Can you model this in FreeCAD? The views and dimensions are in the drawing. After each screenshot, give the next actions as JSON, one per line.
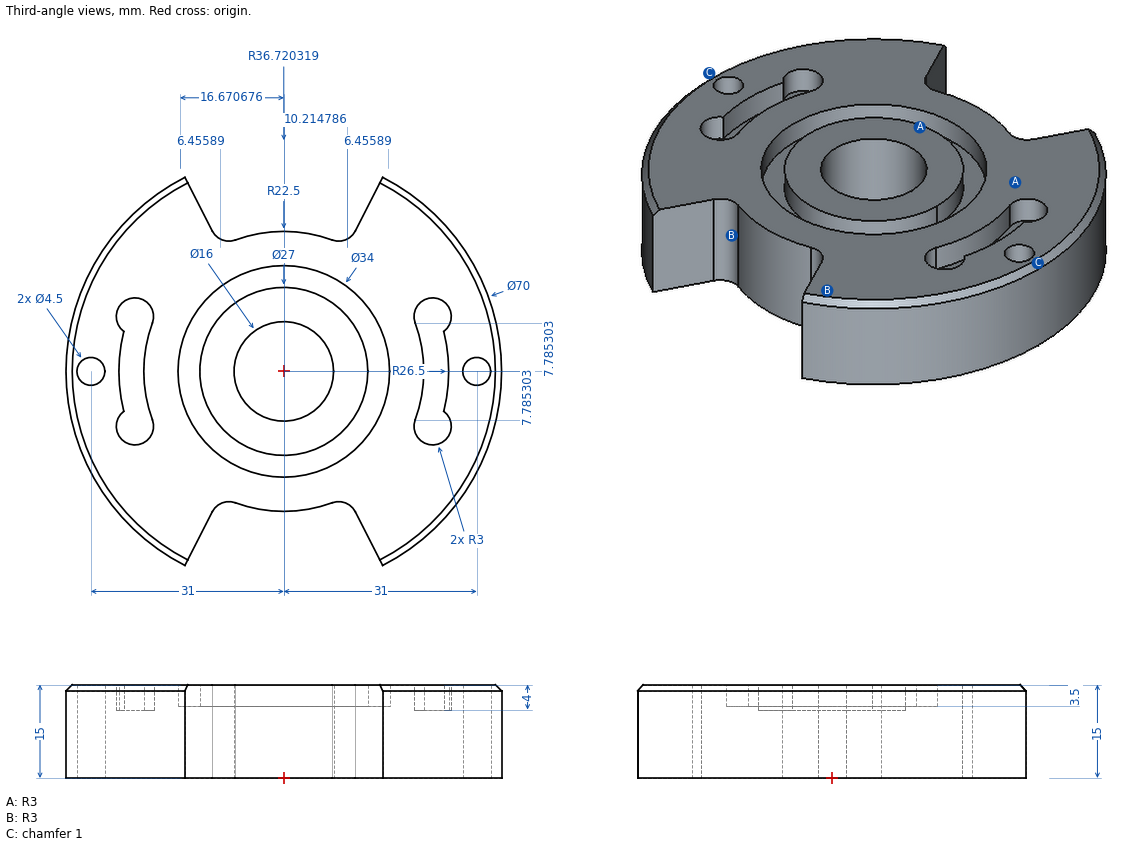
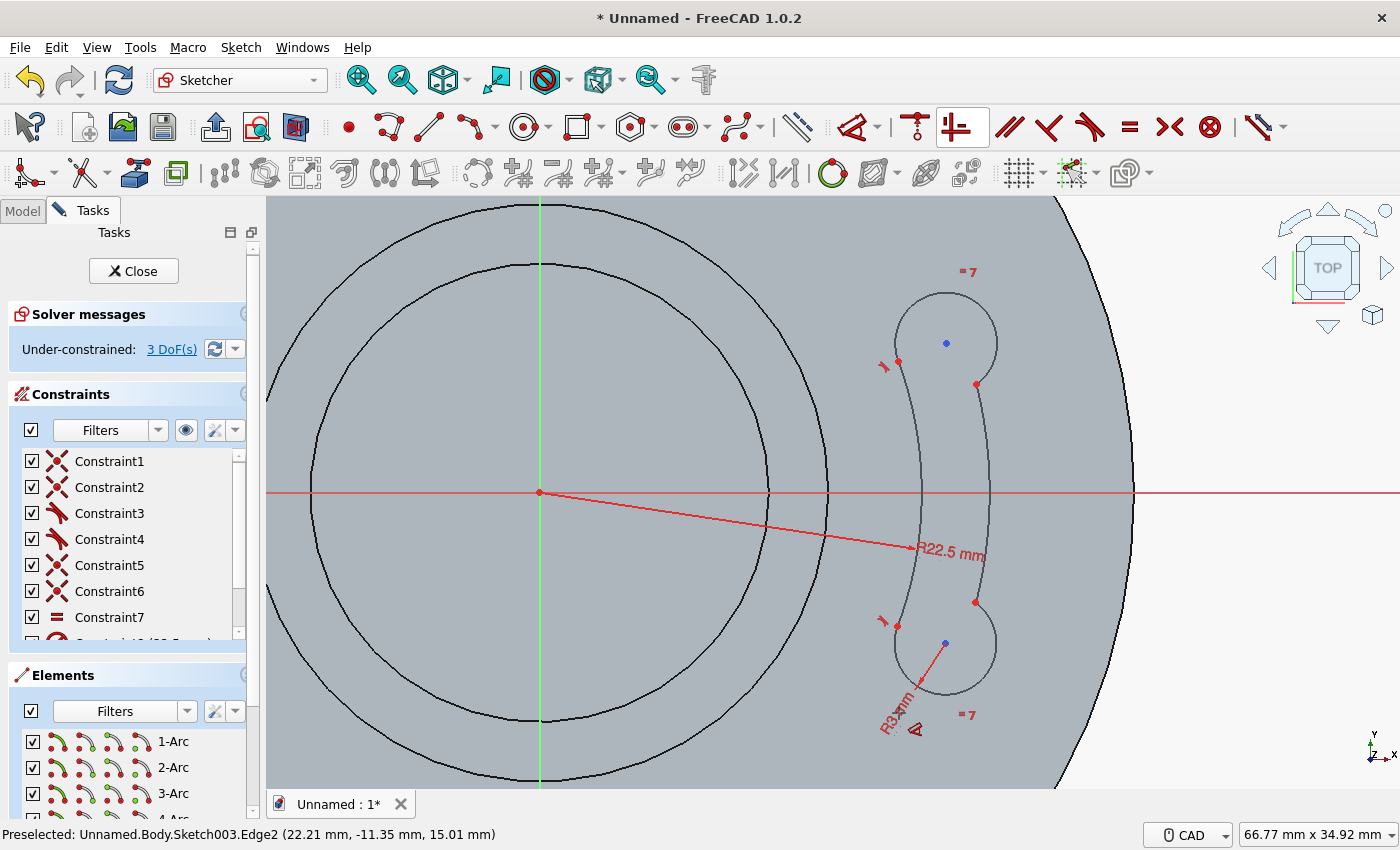
{"action": "left_click", "coordinate": [987, 538]}
{"action": "left_click", "coordinate": [1042, 544]}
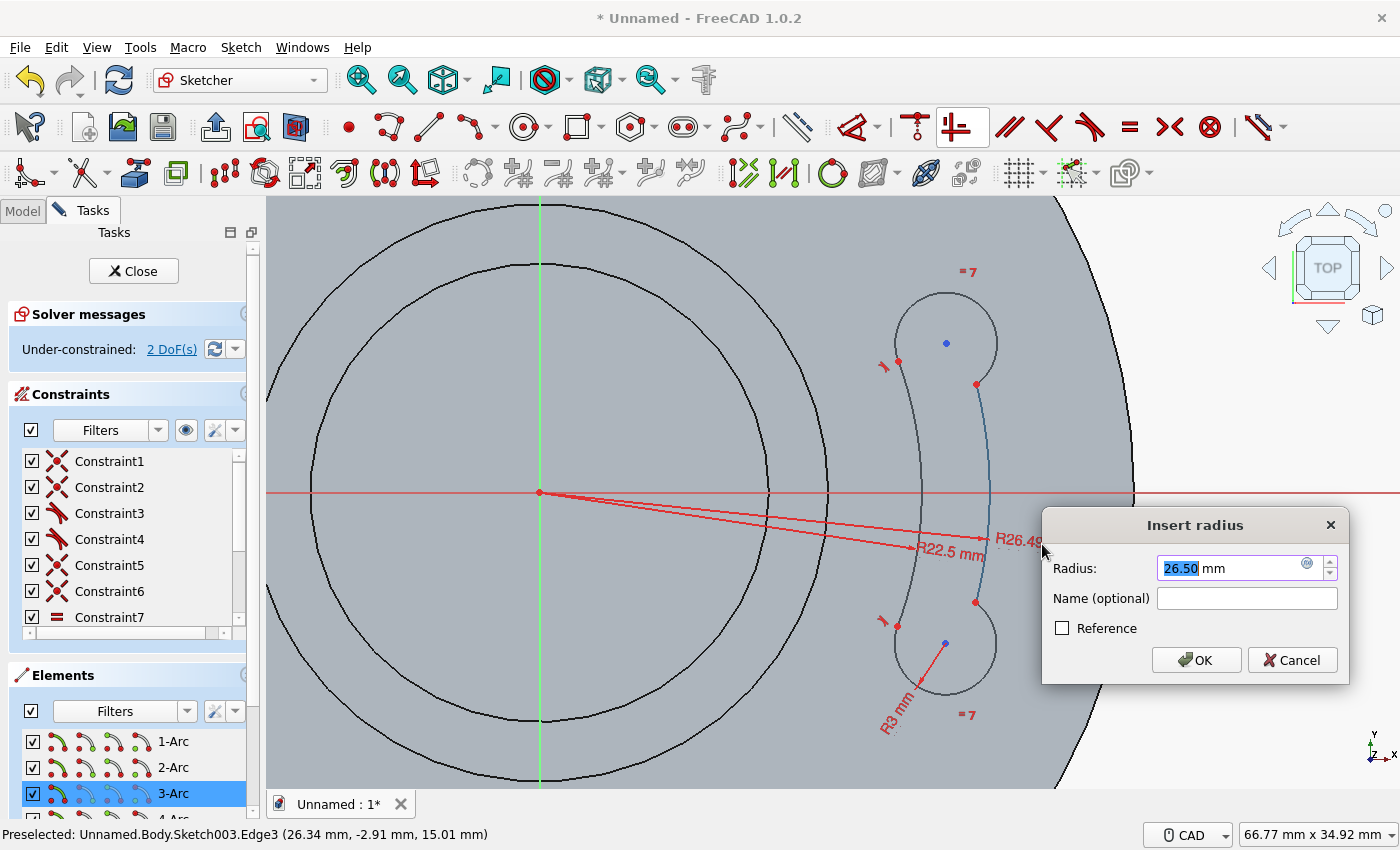
{"action": "type", "text": "26.5"}
{"action": "key", "text": "Return"}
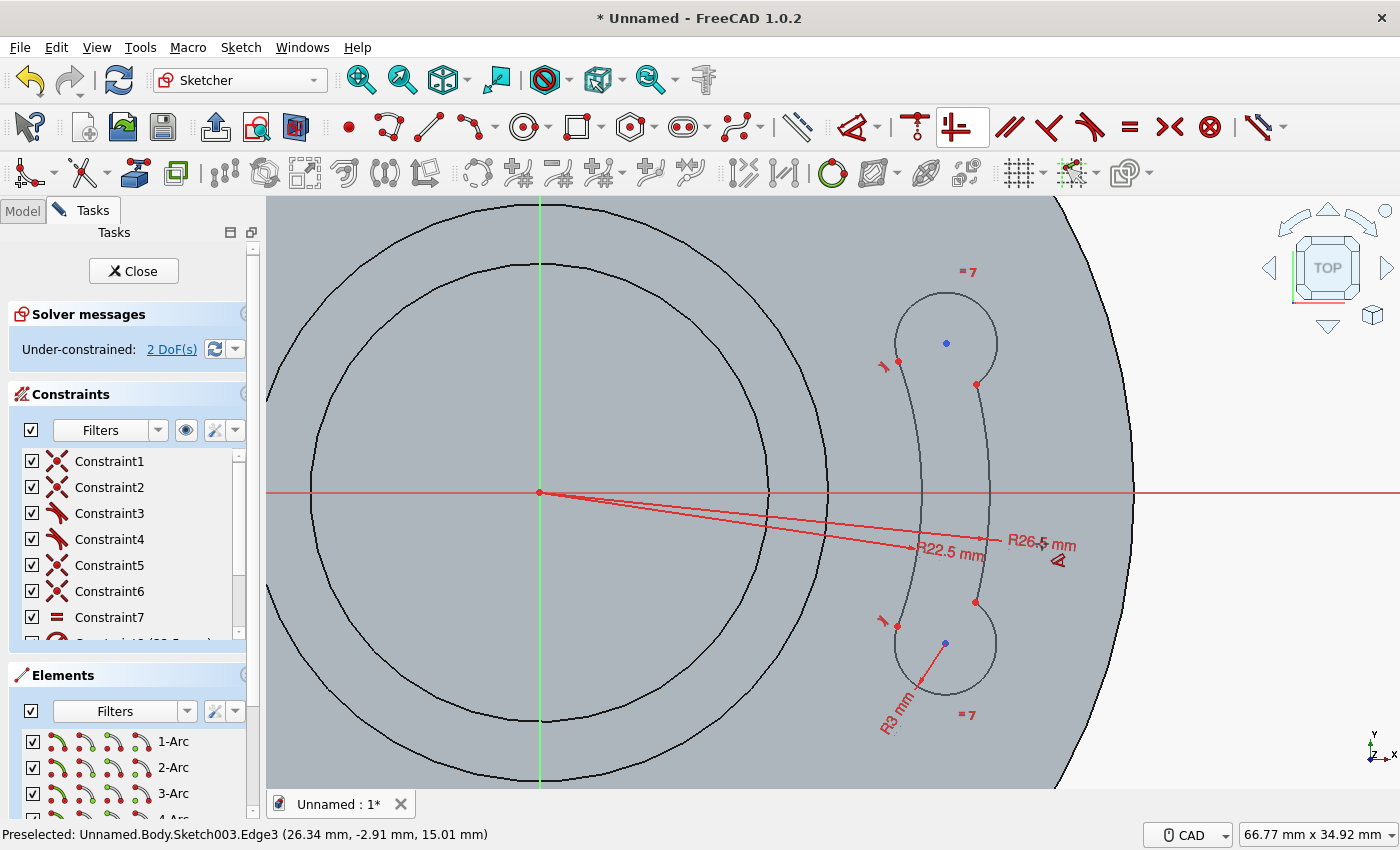
{"action": "left_click", "coordinate": [898, 626]}
{"action": "left_click", "coordinate": [506, 559]}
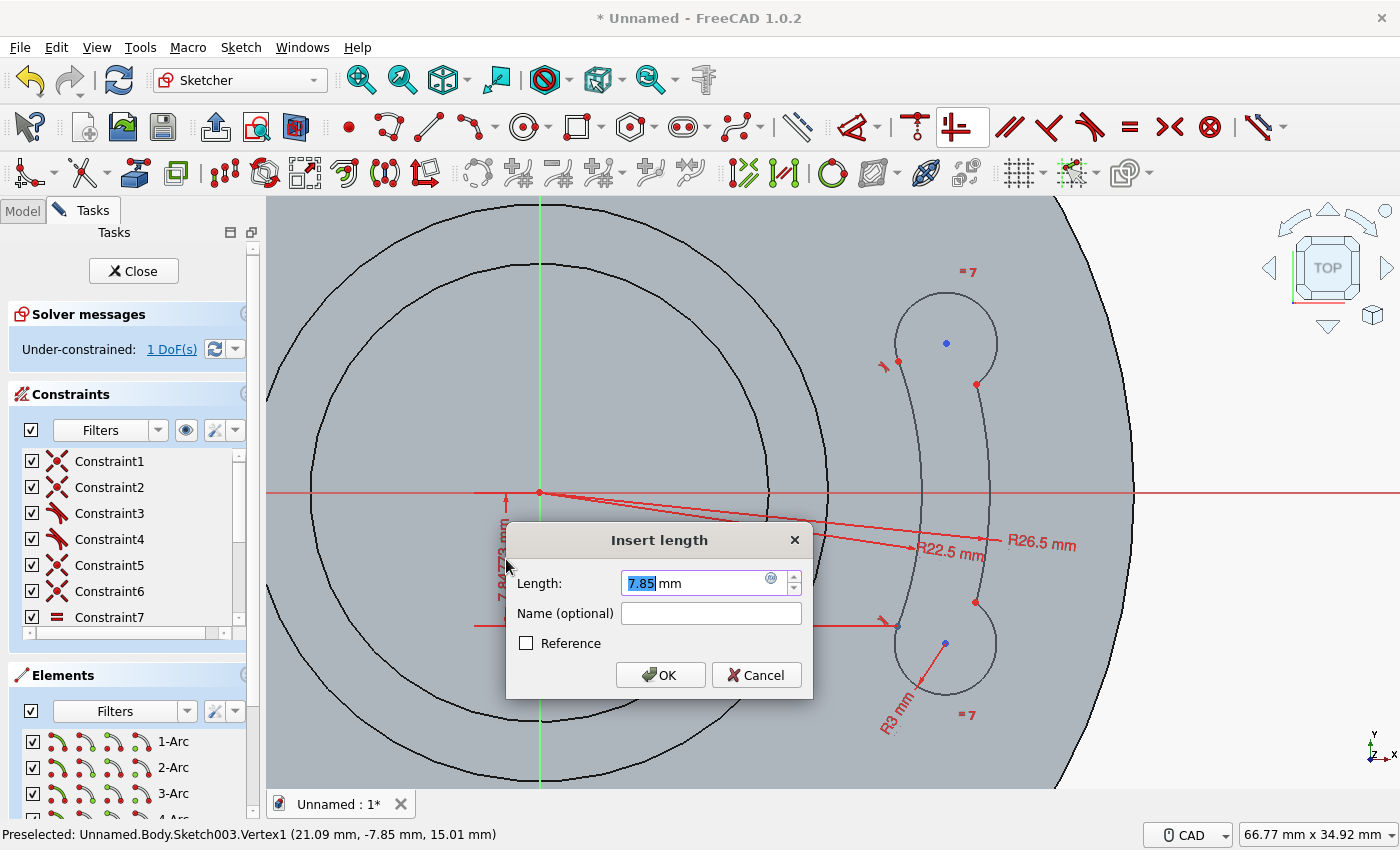
{"action": "type", "text": "7.785303"}
{"action": "key", "text": "Return"}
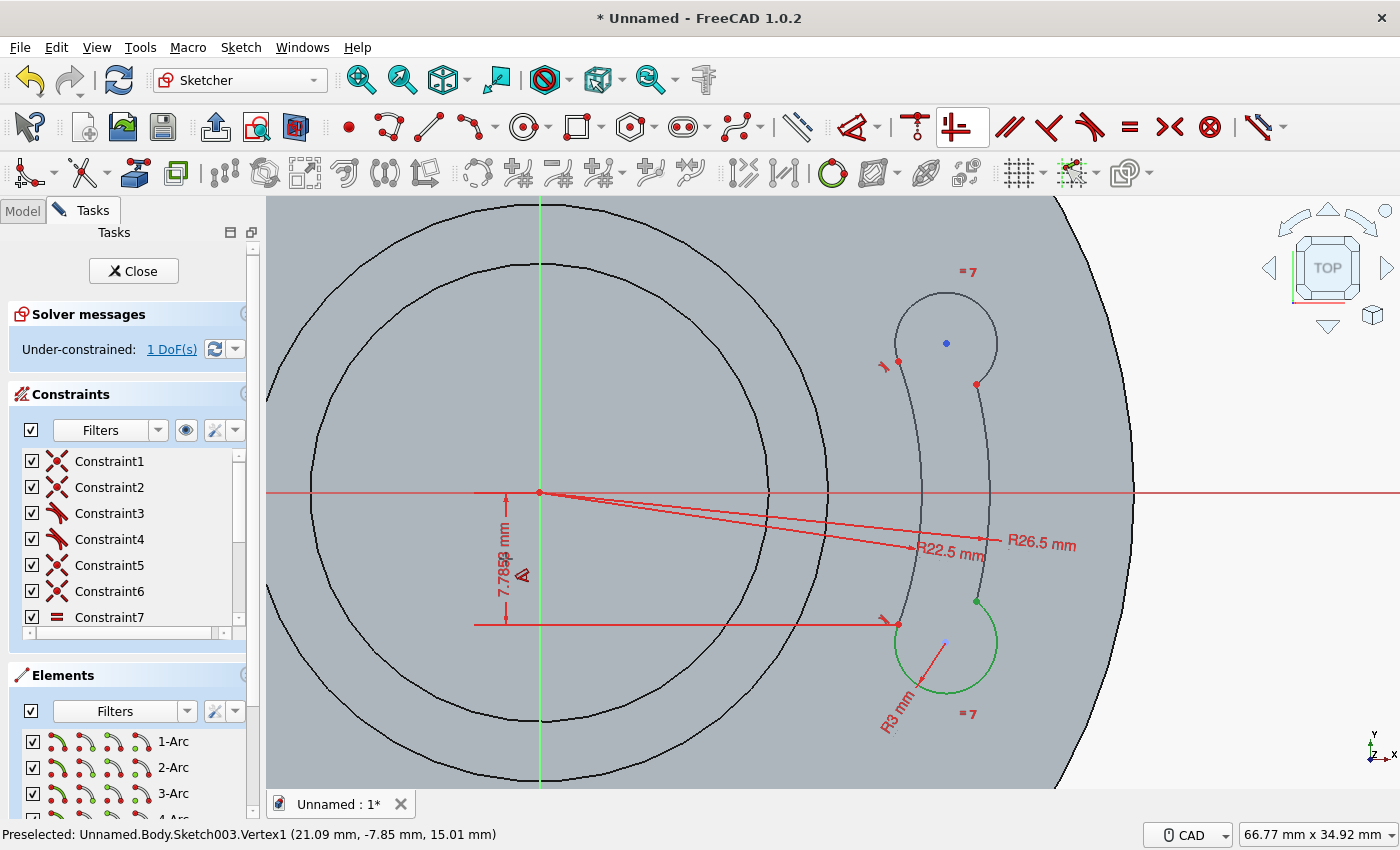
{"action": "left_click", "coordinate": [898, 361]}
{"action": "left_click", "coordinate": [506, 427]}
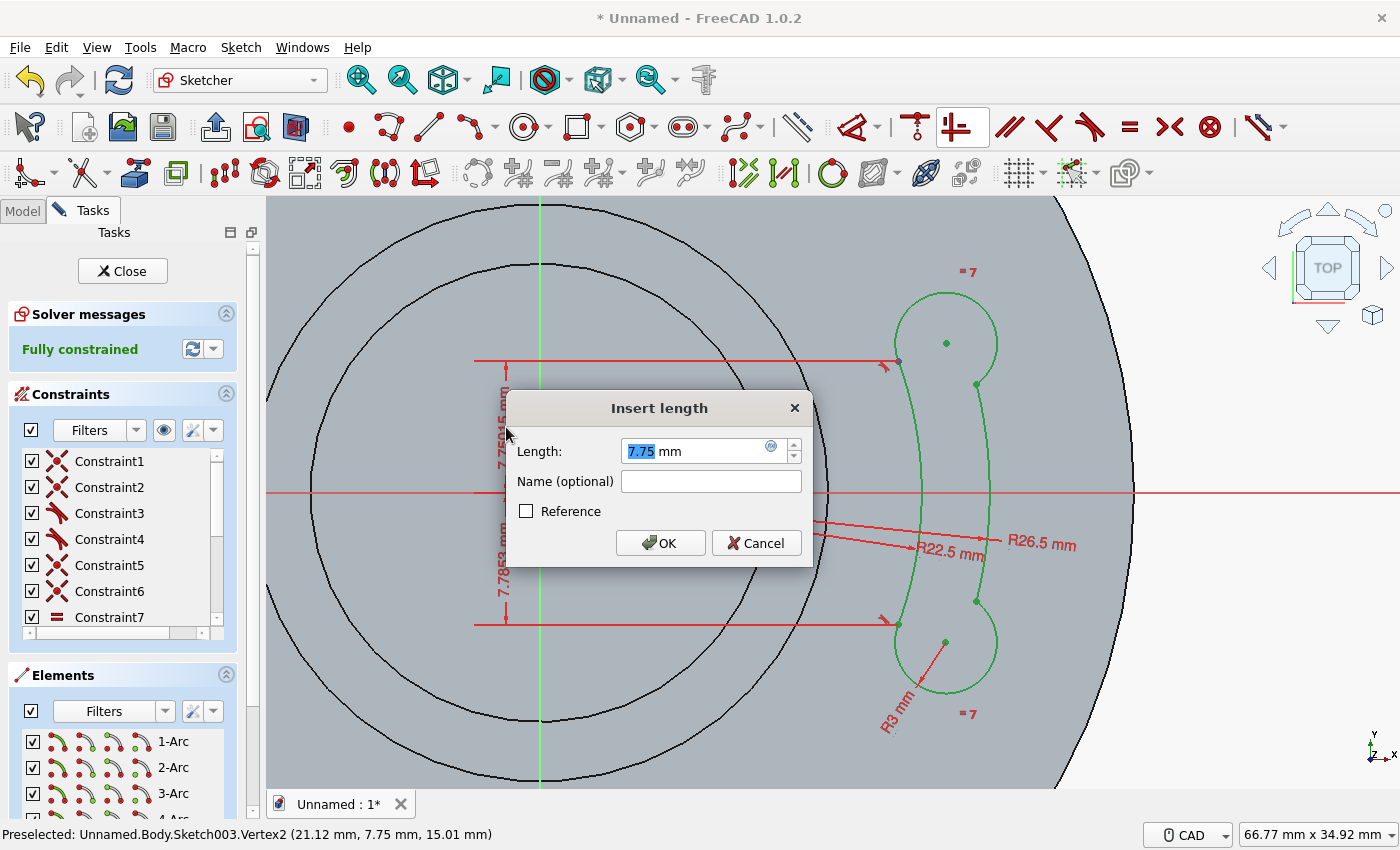
{"action": "type", "text": "7.785303"}
{"action": "key", "text": "Return"}
{"action": "key", "text": "Escape"}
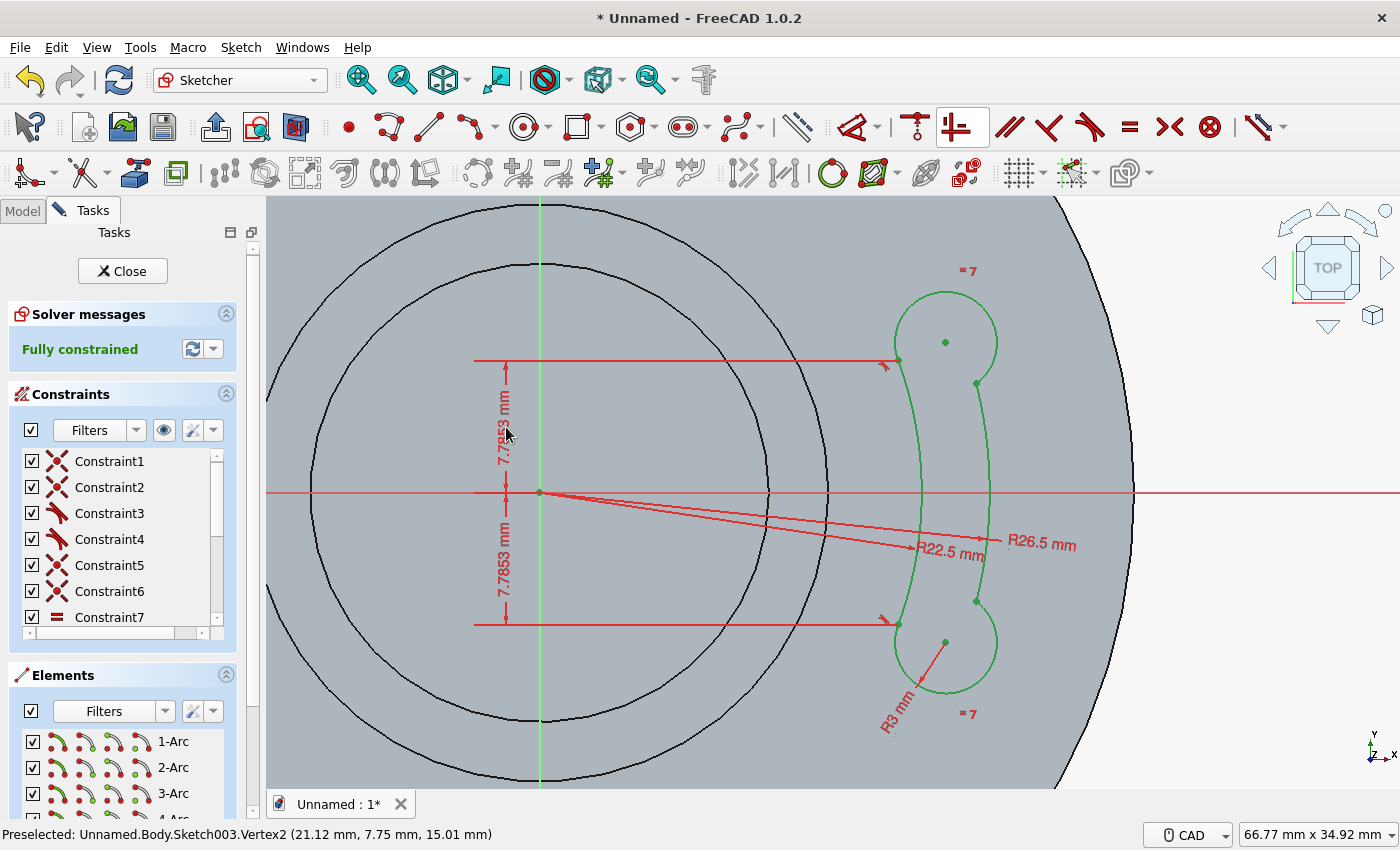
{"action": "left_click", "coordinate": [123, 271]}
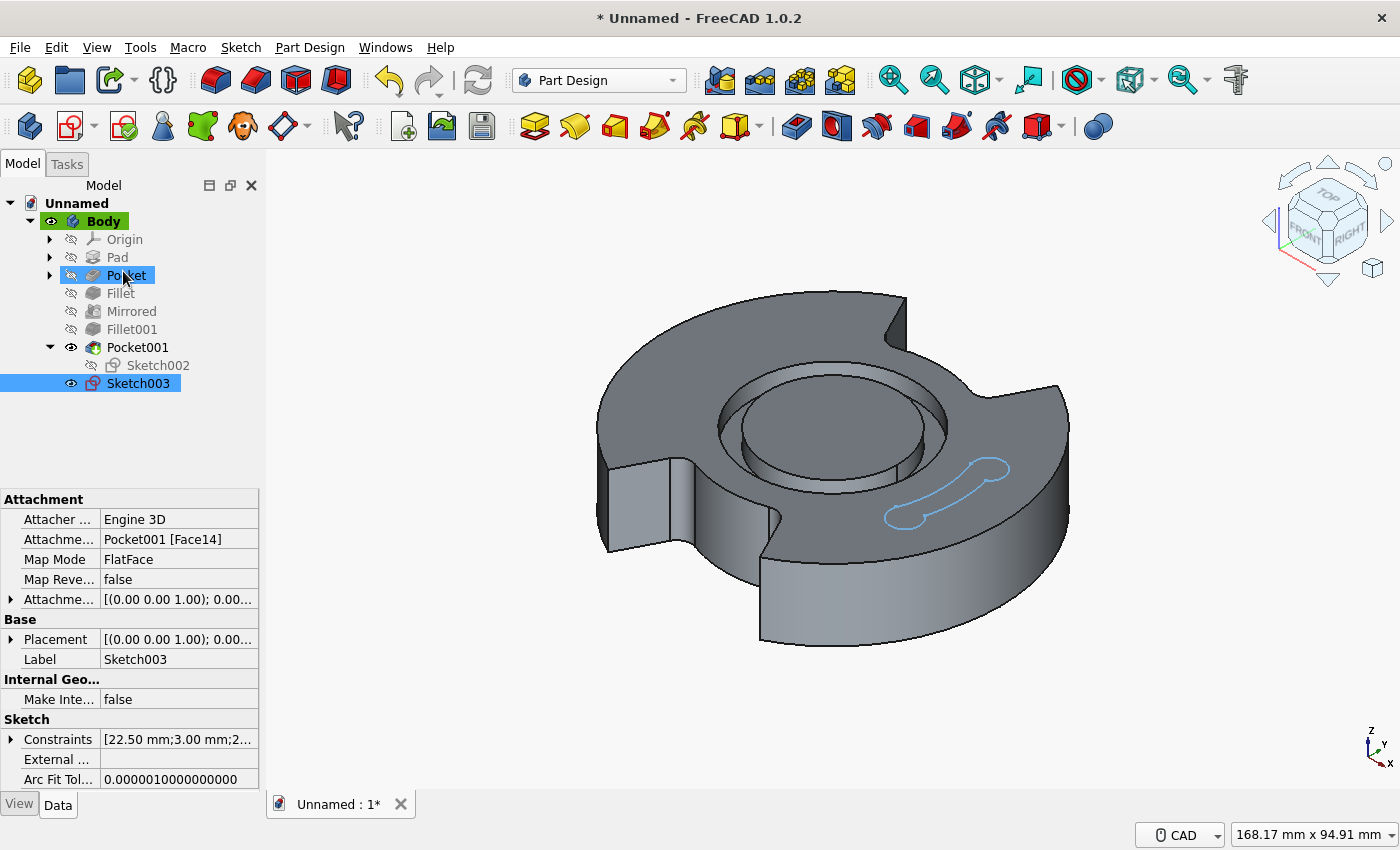
{"action": "left_click", "coordinate": [798, 126]}